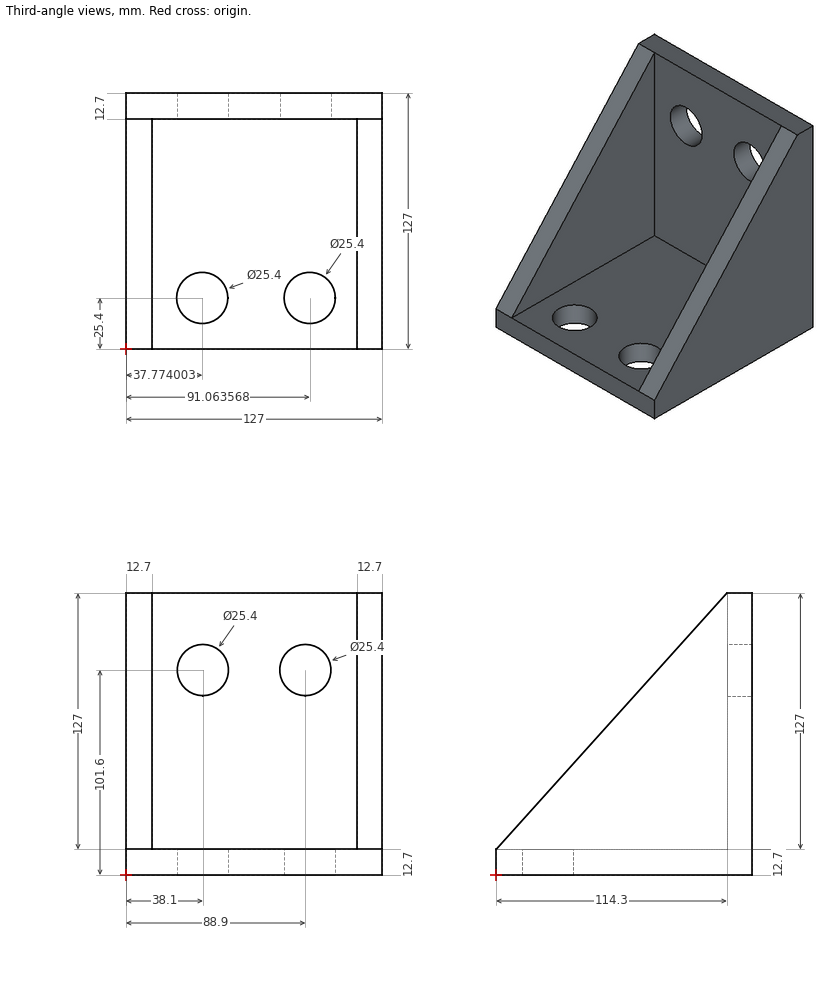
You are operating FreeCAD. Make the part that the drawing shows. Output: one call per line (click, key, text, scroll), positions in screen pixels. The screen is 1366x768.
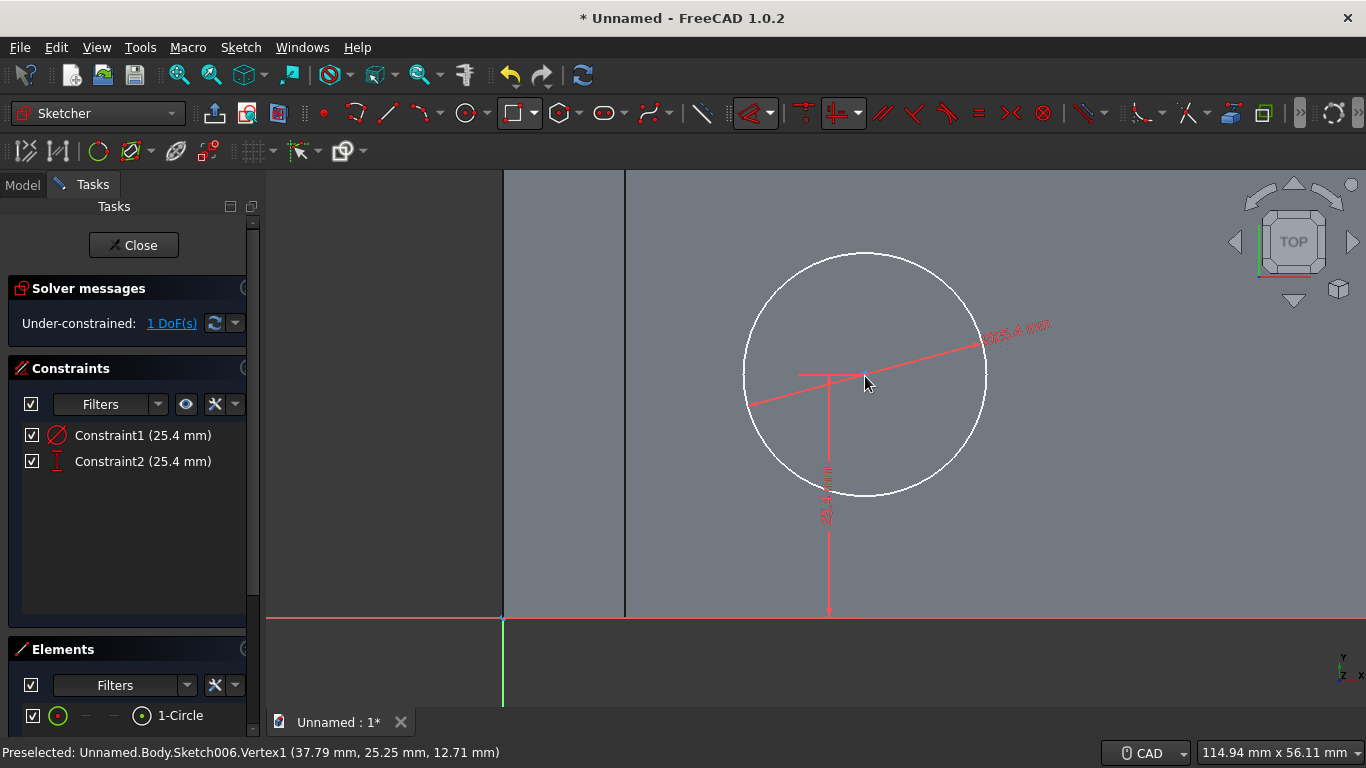
click(865, 375)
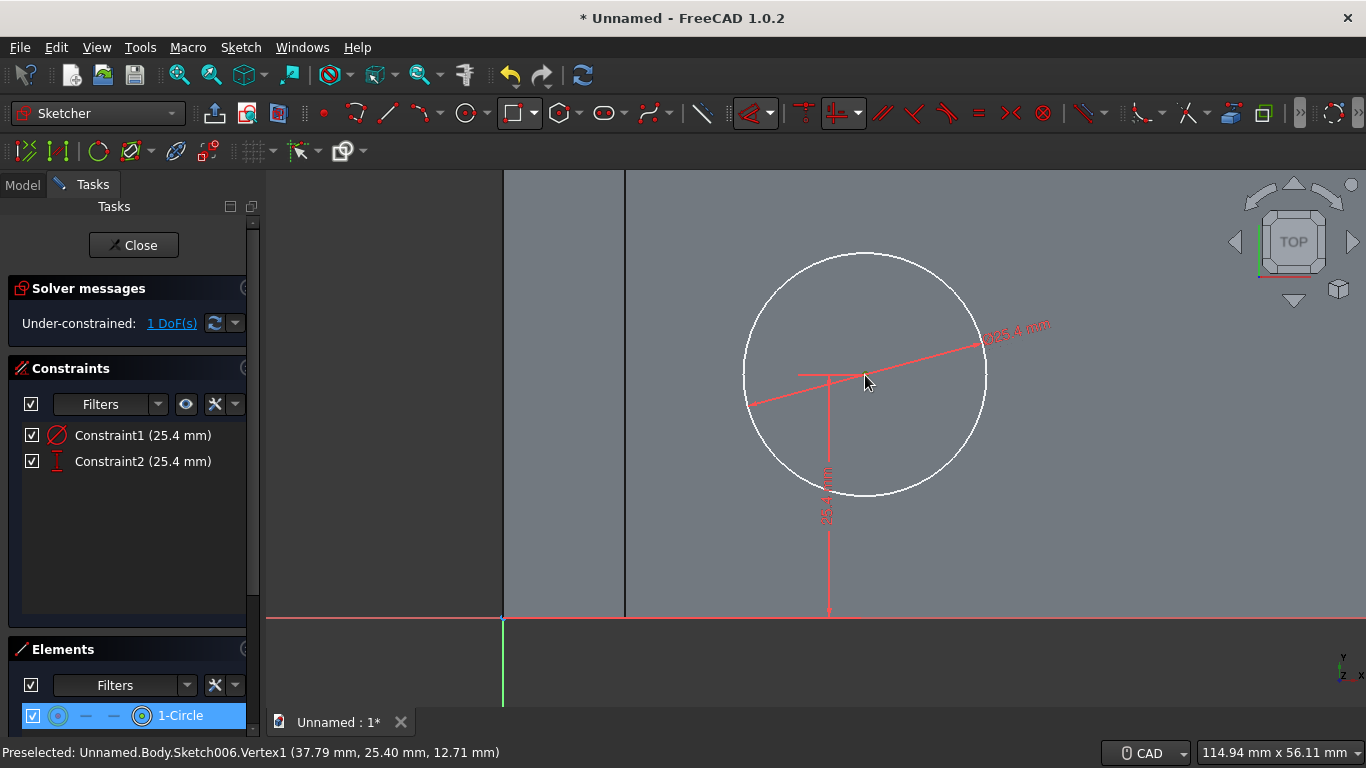
click(772, 114)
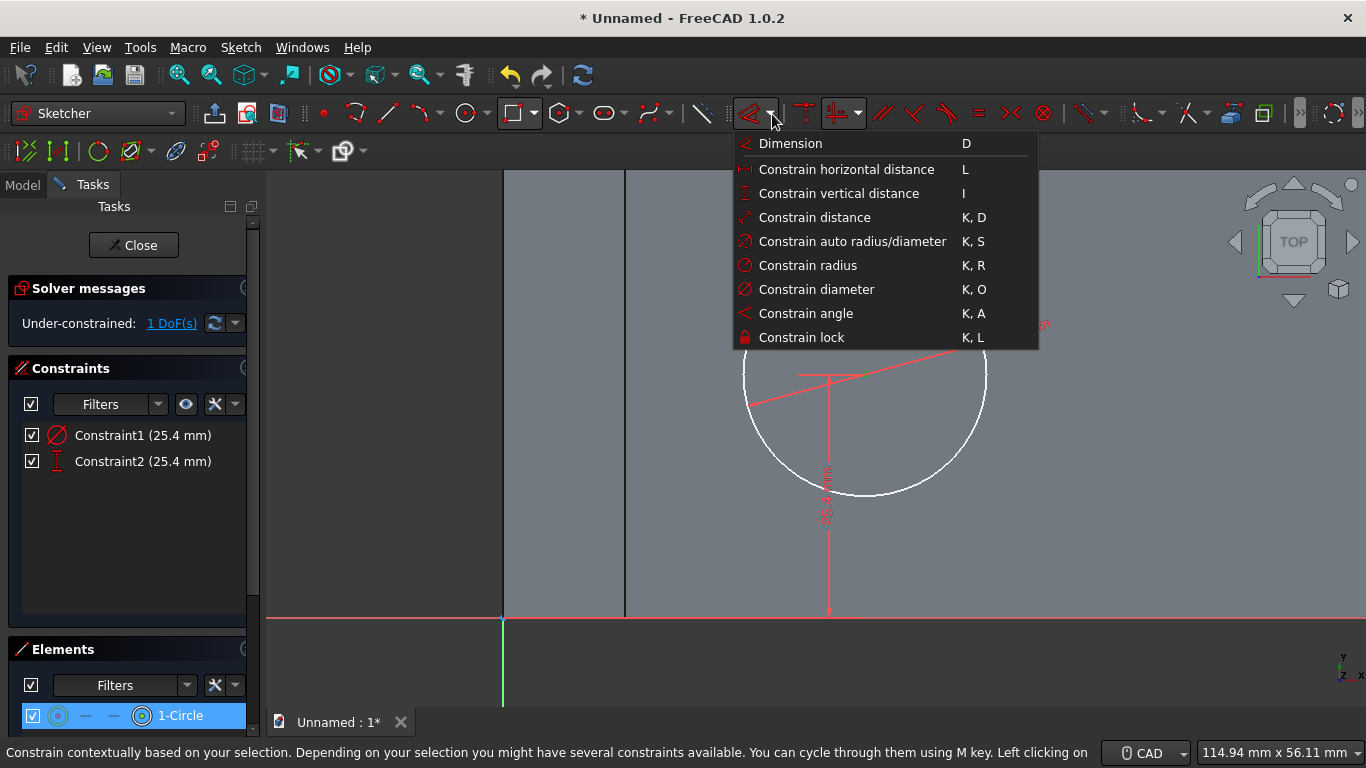
click(886, 169)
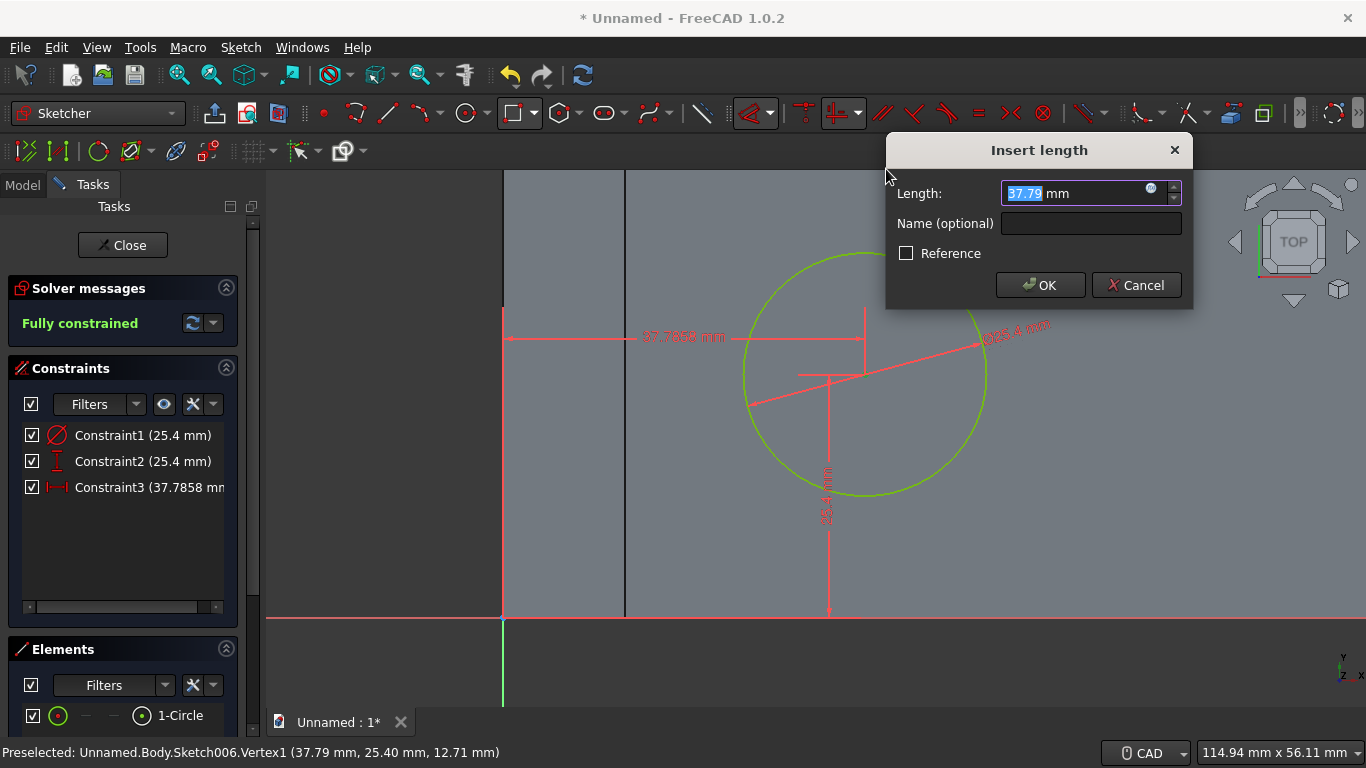
text(37.774003)
key(Return)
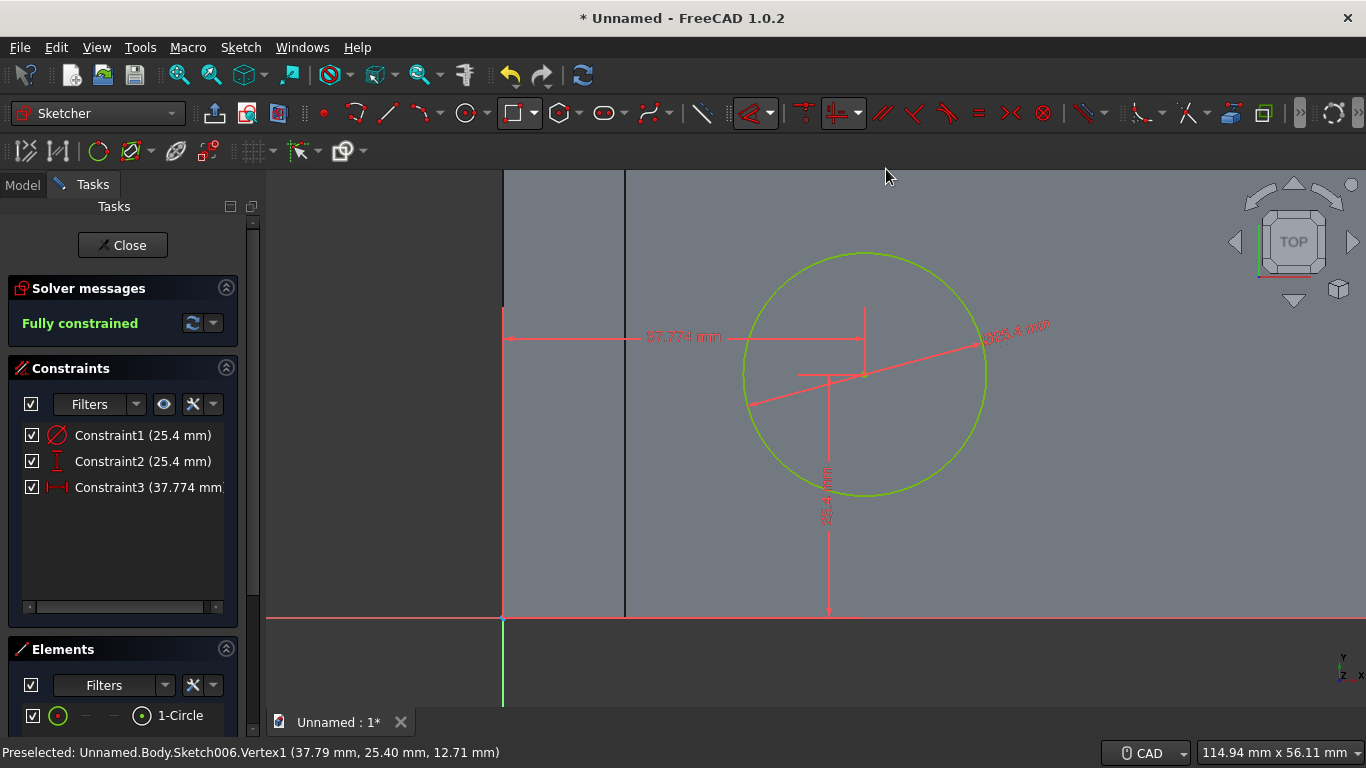
click(123, 245)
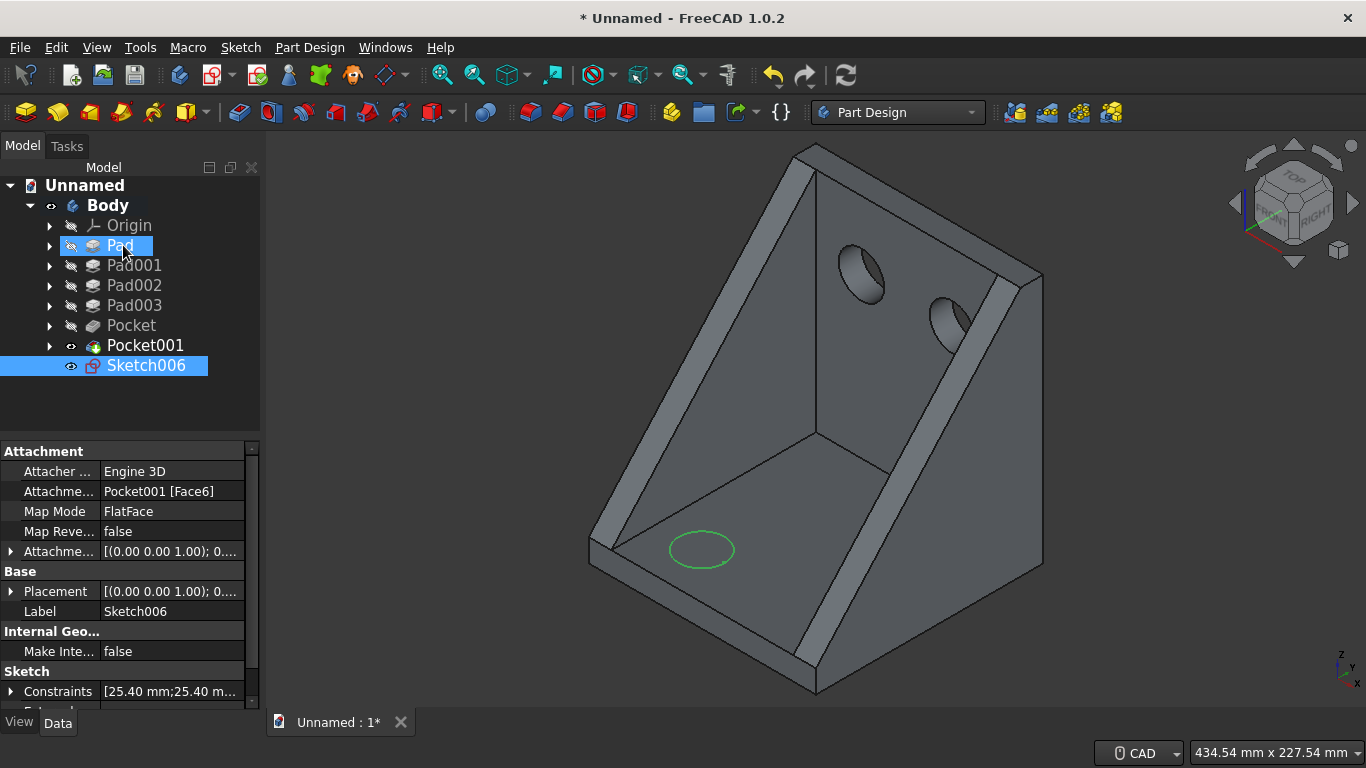
click(240, 112)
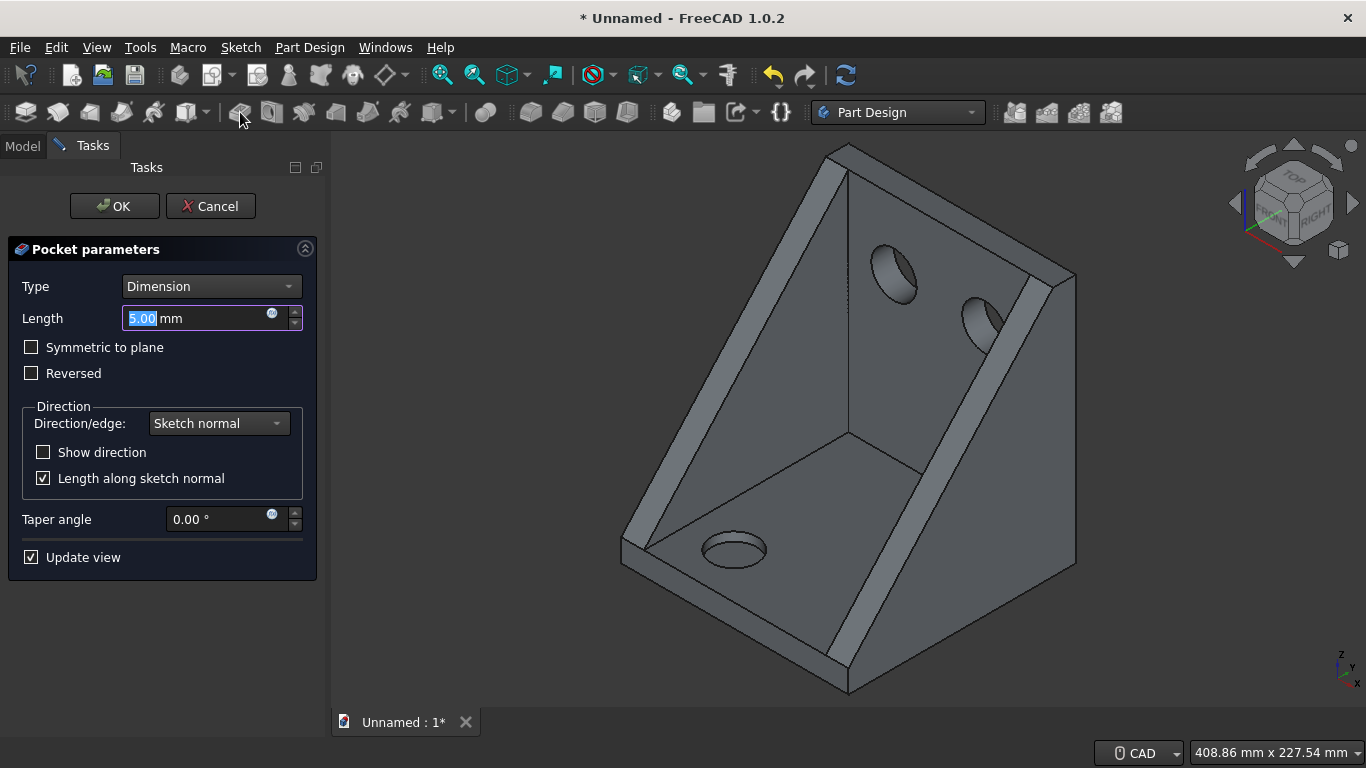
text(12.7)
key(Tab)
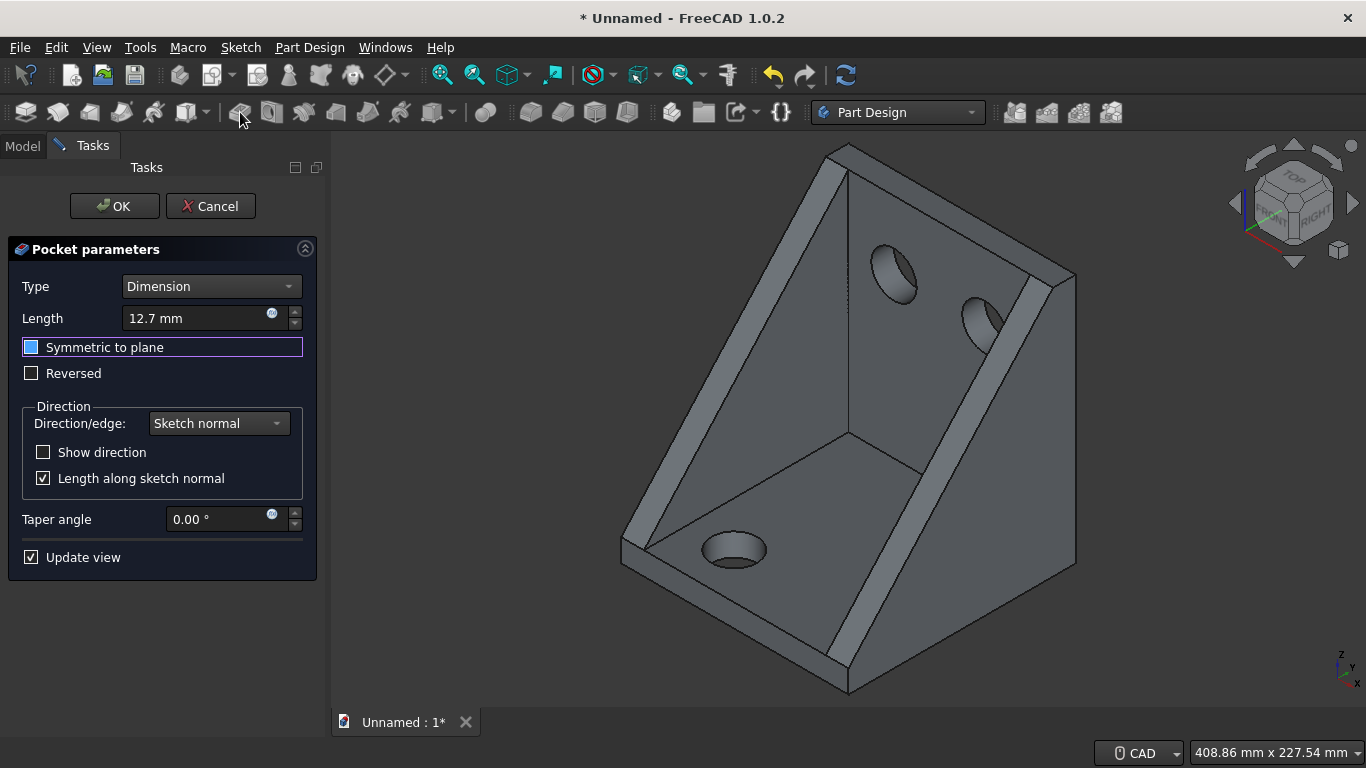
click(115, 206)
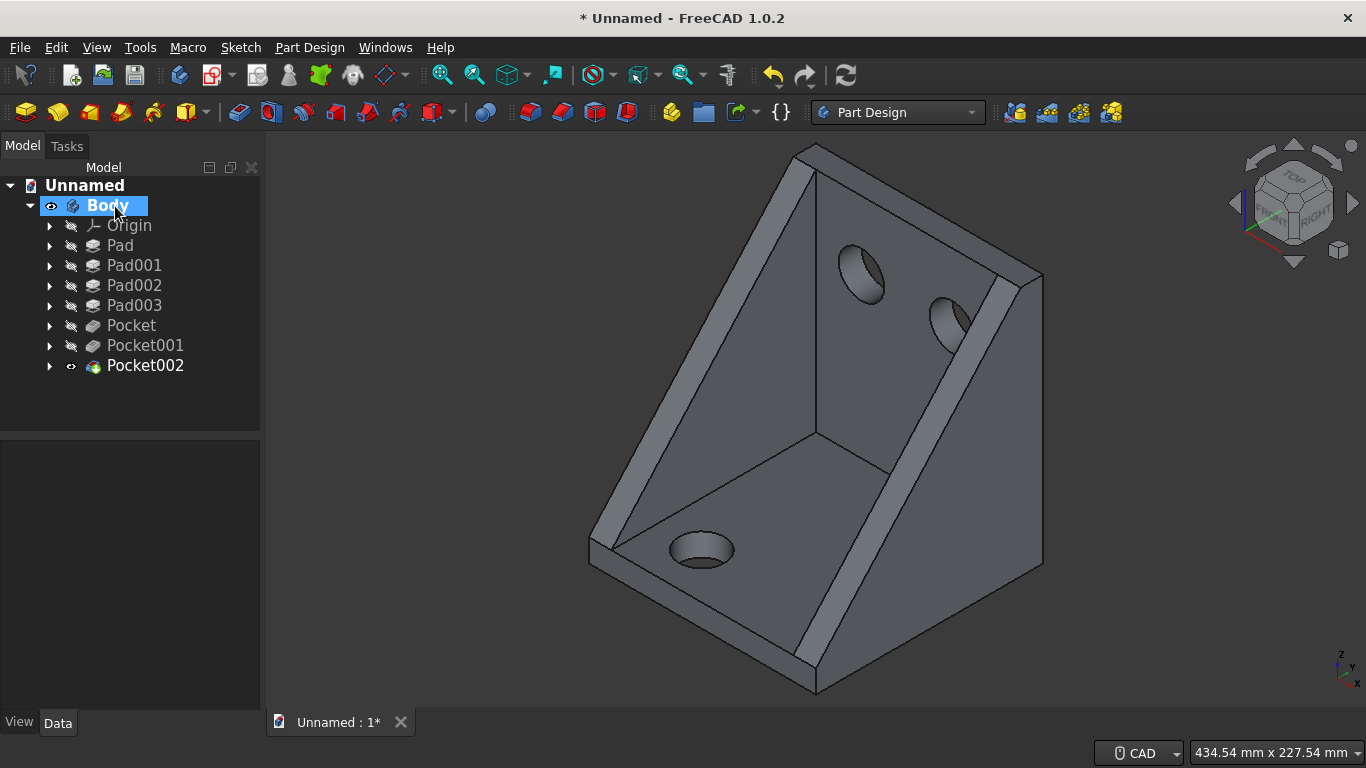
click(834, 526)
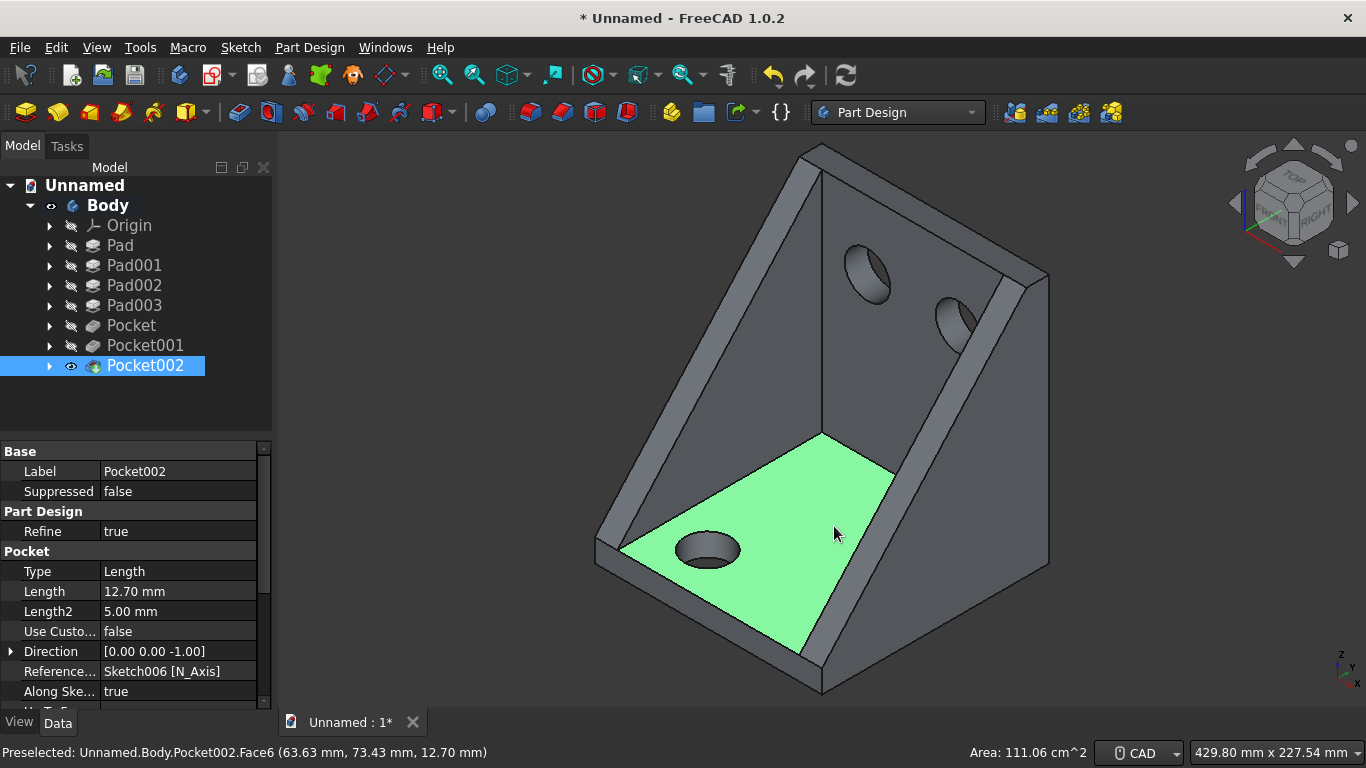
click(212, 76)